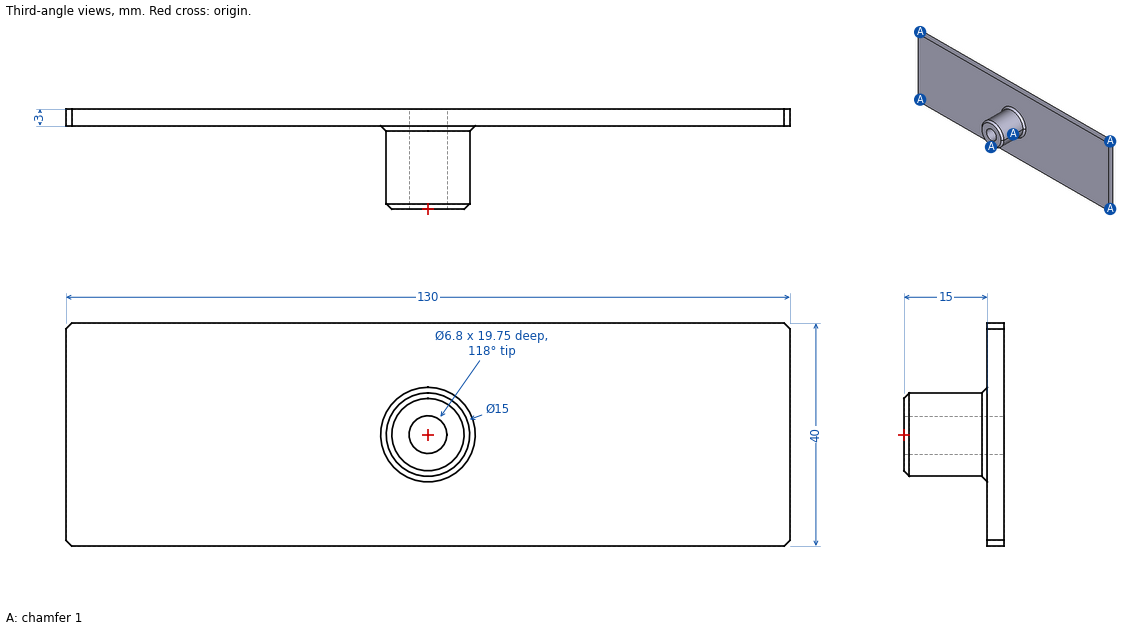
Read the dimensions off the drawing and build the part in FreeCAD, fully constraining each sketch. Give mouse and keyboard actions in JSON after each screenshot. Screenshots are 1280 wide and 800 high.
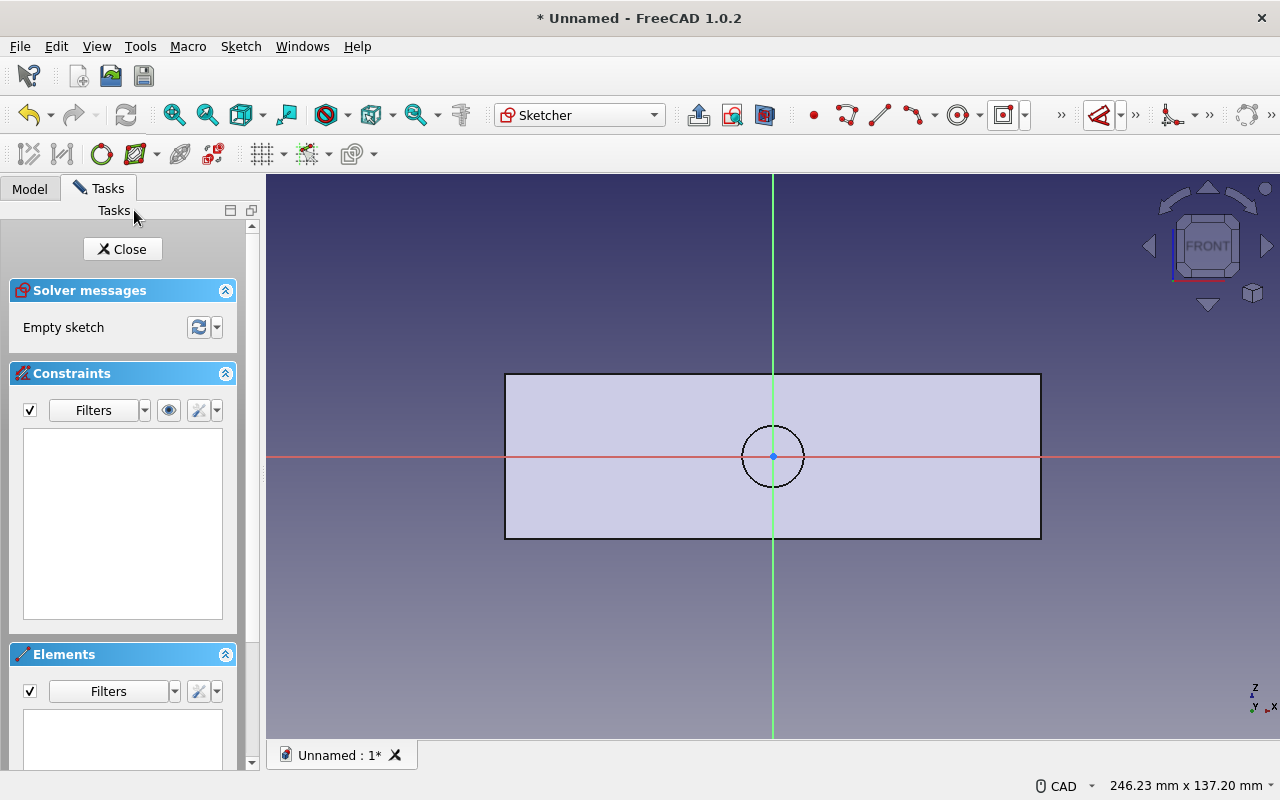
{"action": "scroll", "coordinate": [778, 457], "scroll_direction": "up", "scroll_amount": 13}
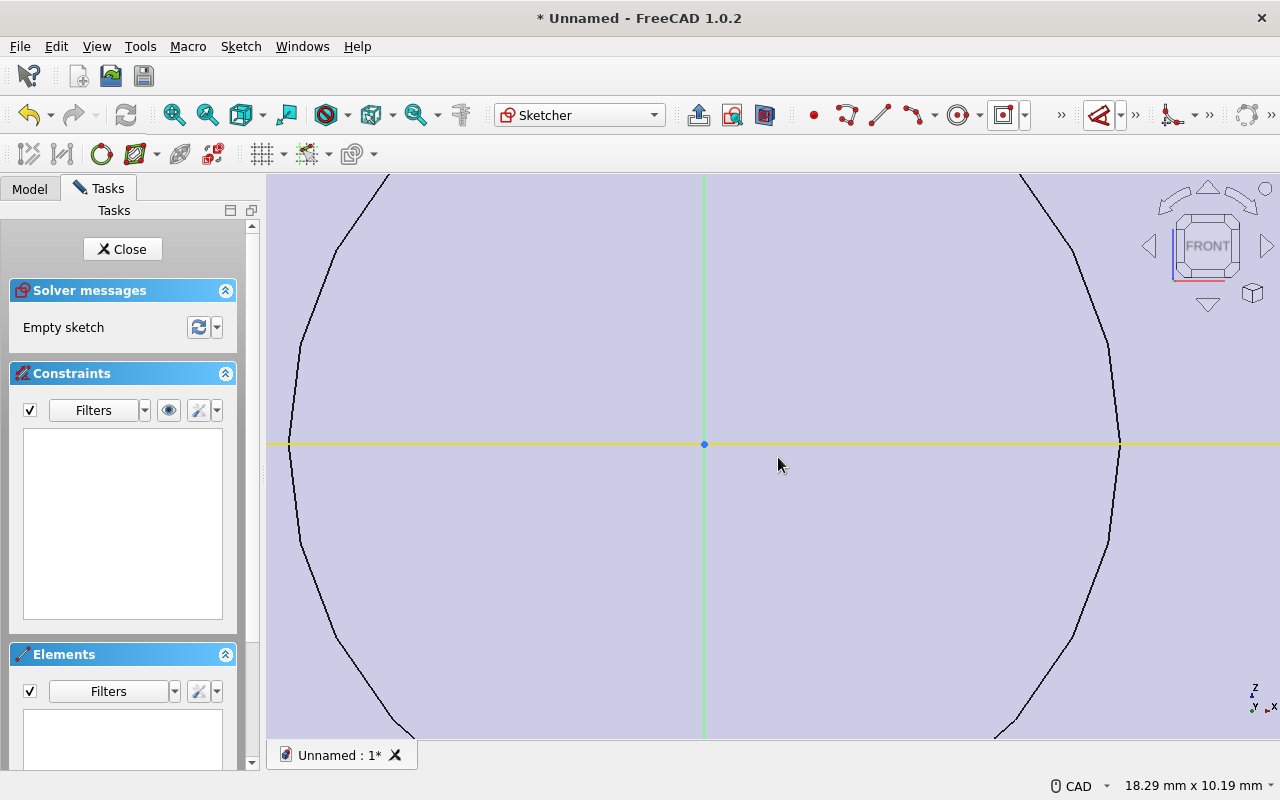
{"action": "left_click", "coordinate": [958, 116]}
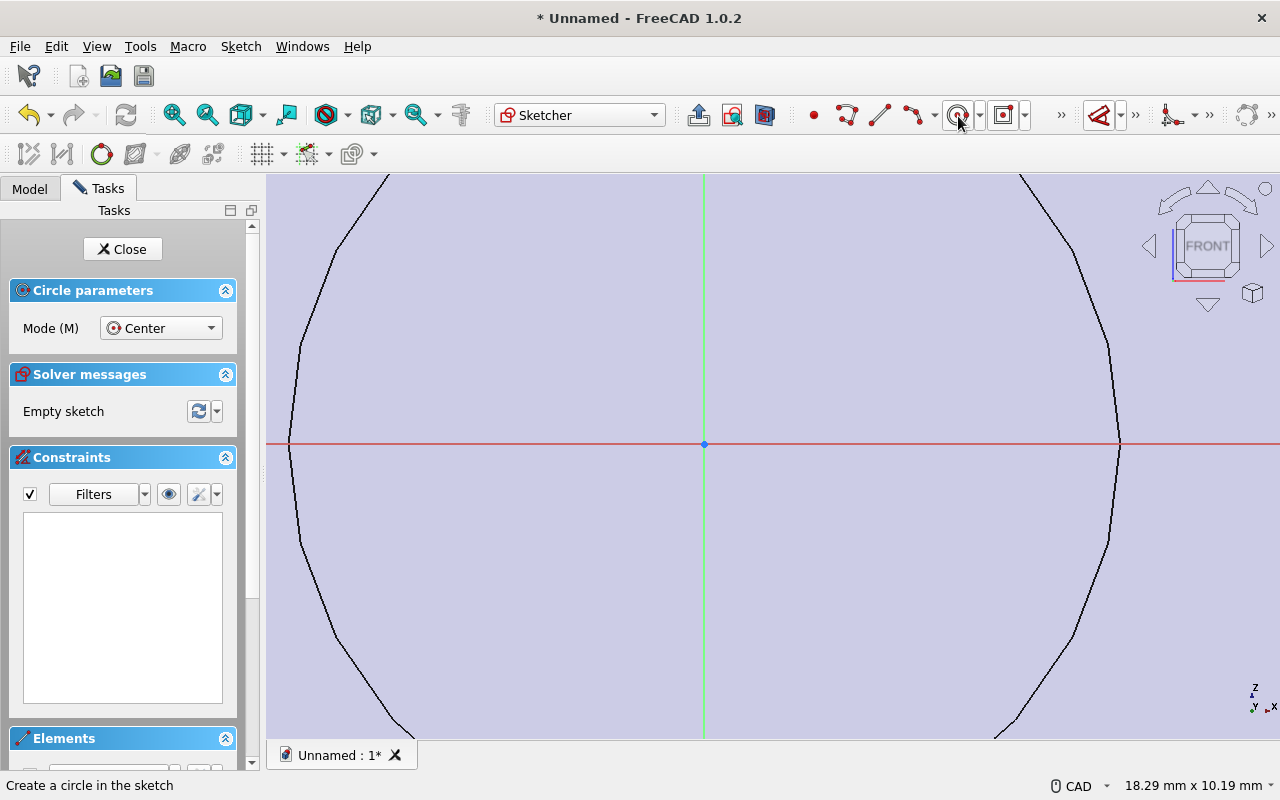
{"action": "left_click", "coordinate": [704, 444]}
{"action": "mouse_move", "coordinate": [838, 311]}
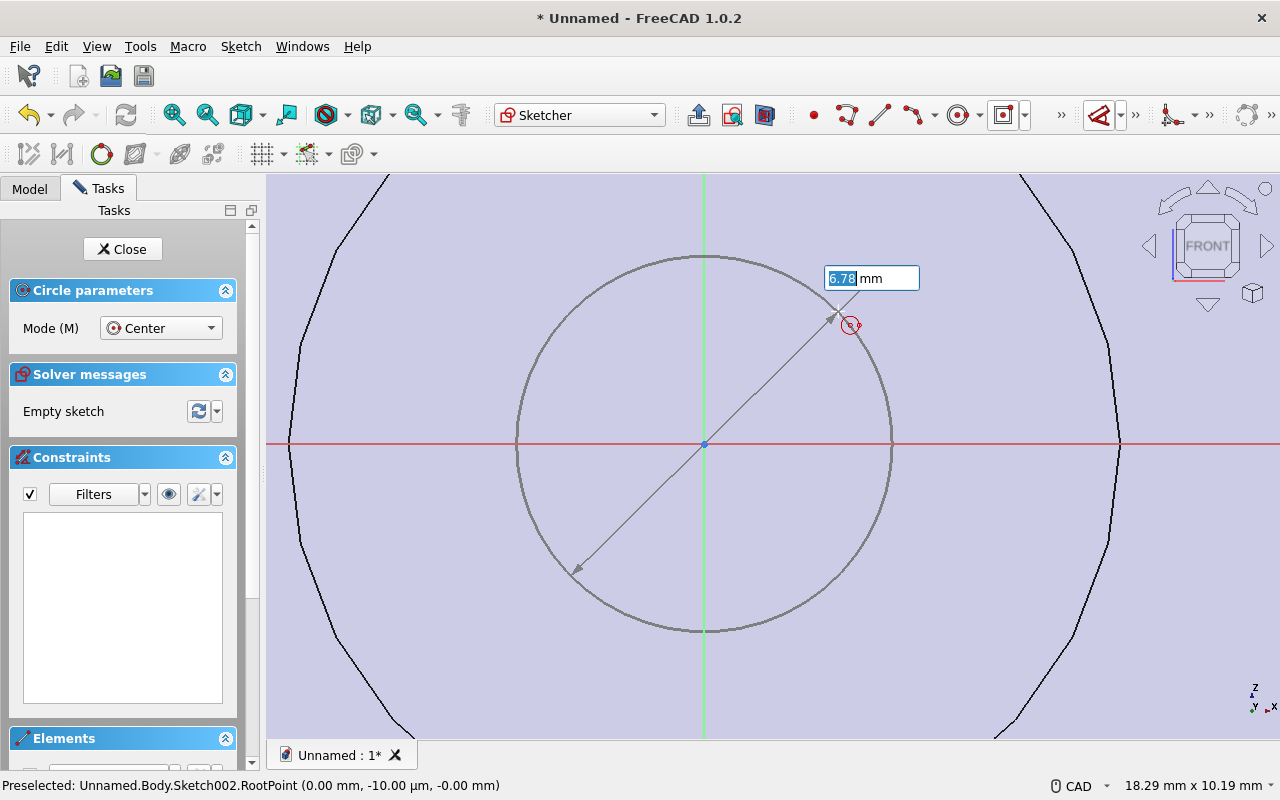
{"action": "type", "text": "6.8"}
{"action": "key", "text": "Return"}
{"action": "key", "text": "Escape"}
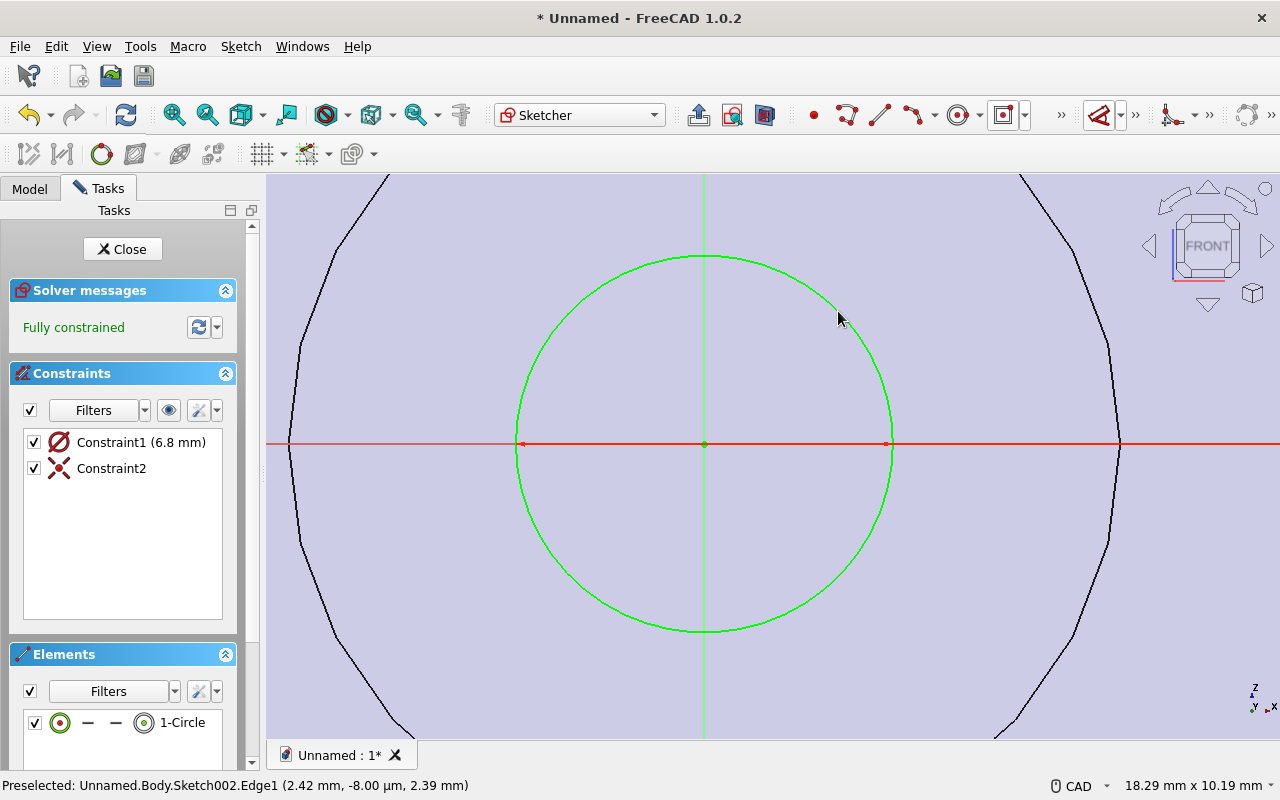
{"action": "left_click", "coordinate": [123, 249]}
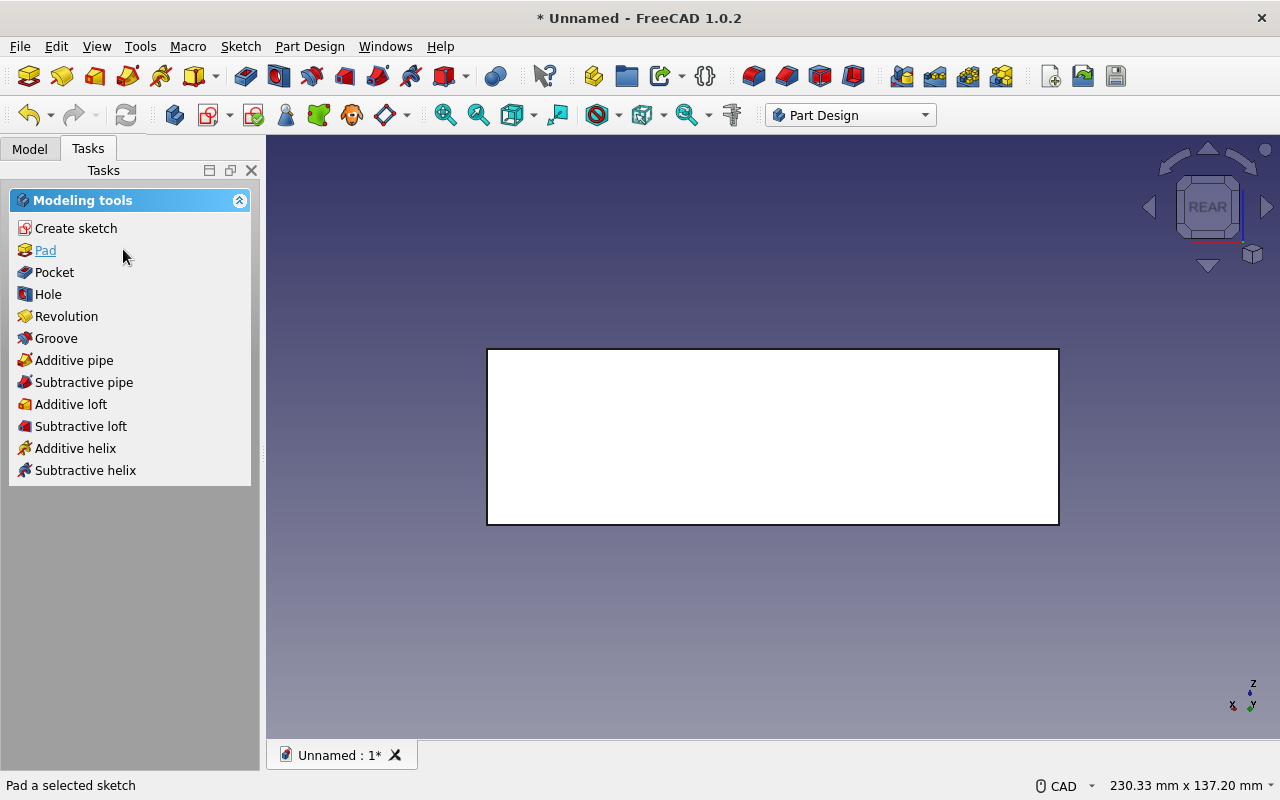
{"action": "left_click", "coordinate": [279, 76]}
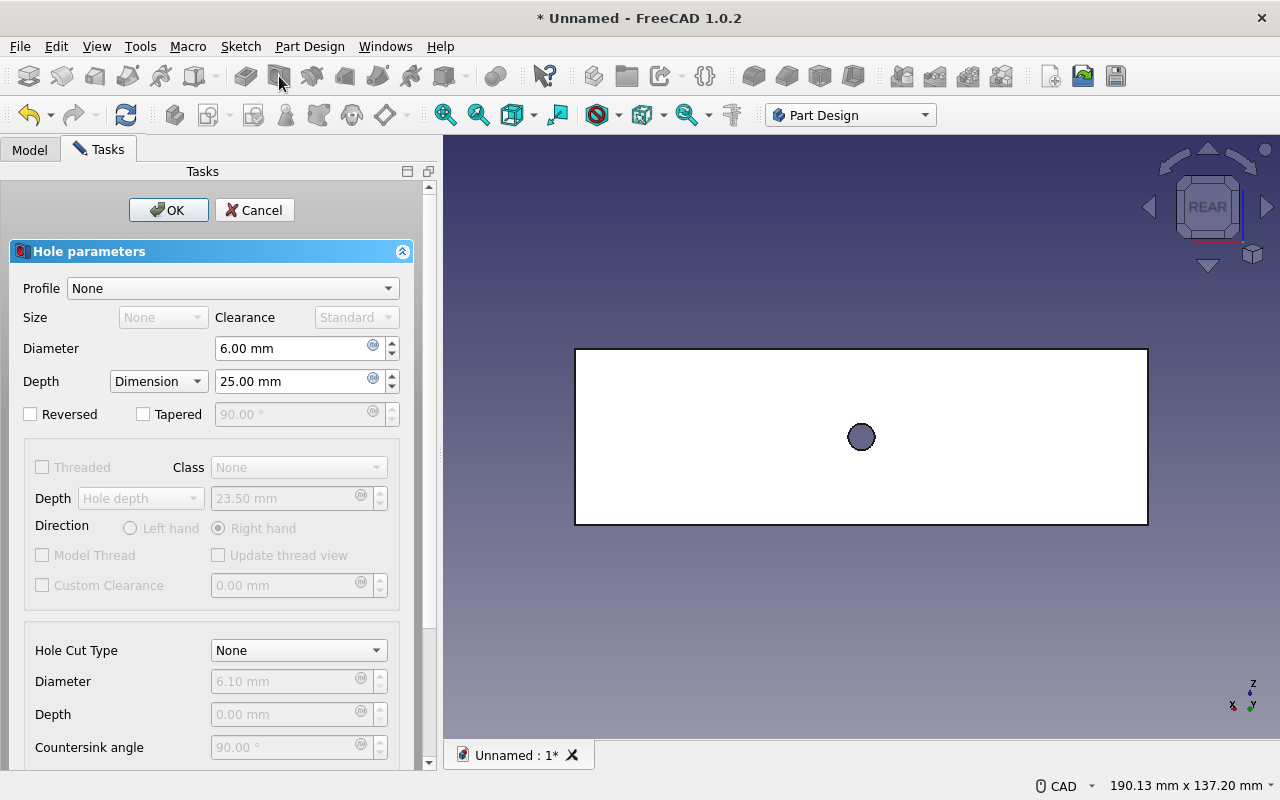
{"action": "triple_click", "coordinate": [300, 348]}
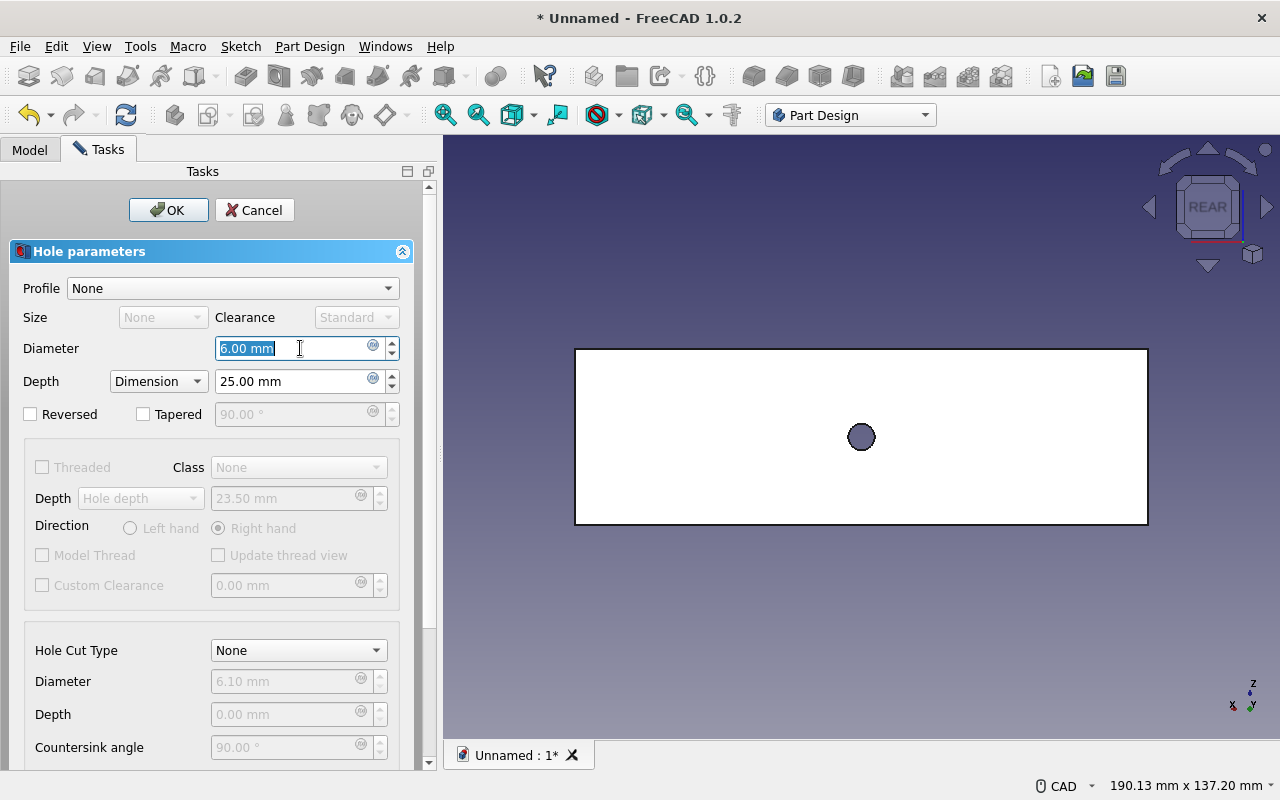
{"action": "type", "text": "6.8"}
{"action": "key", "text": "Tab"}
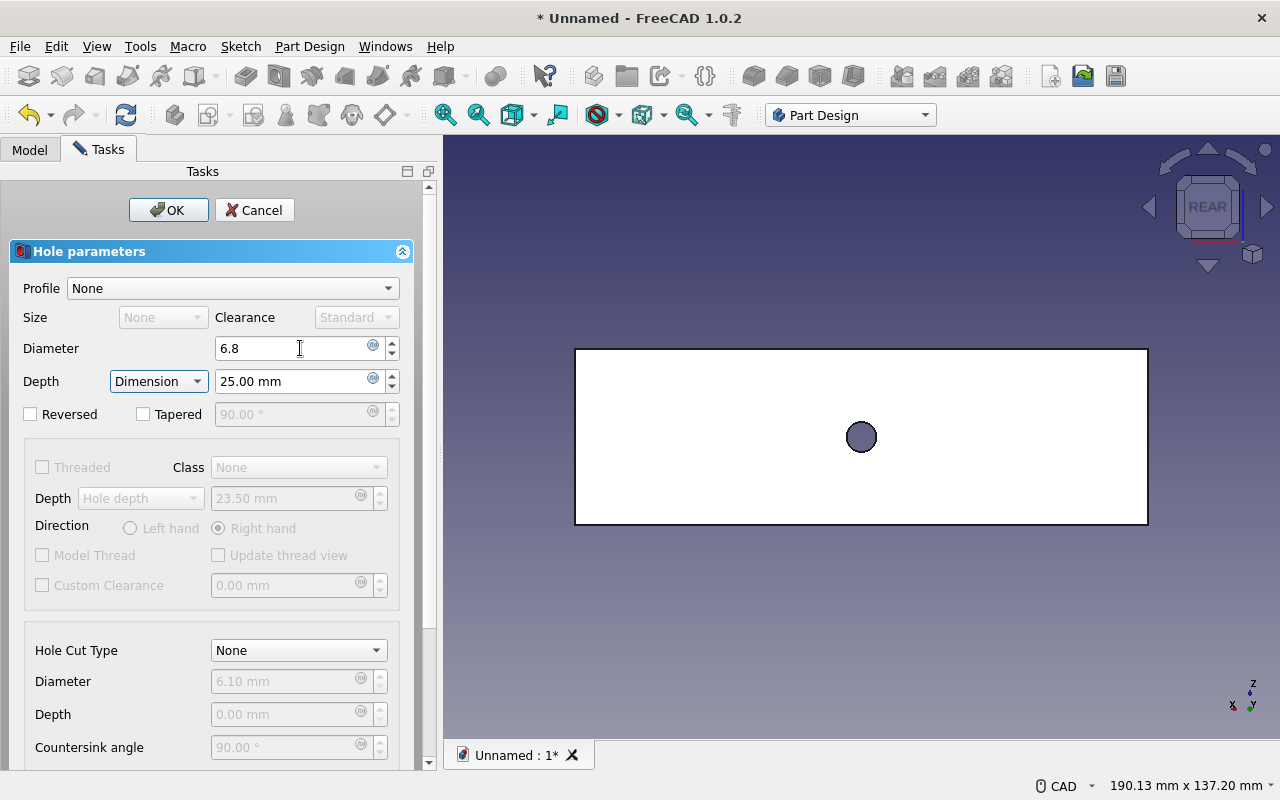
{"action": "triple_click", "coordinate": [300, 382]}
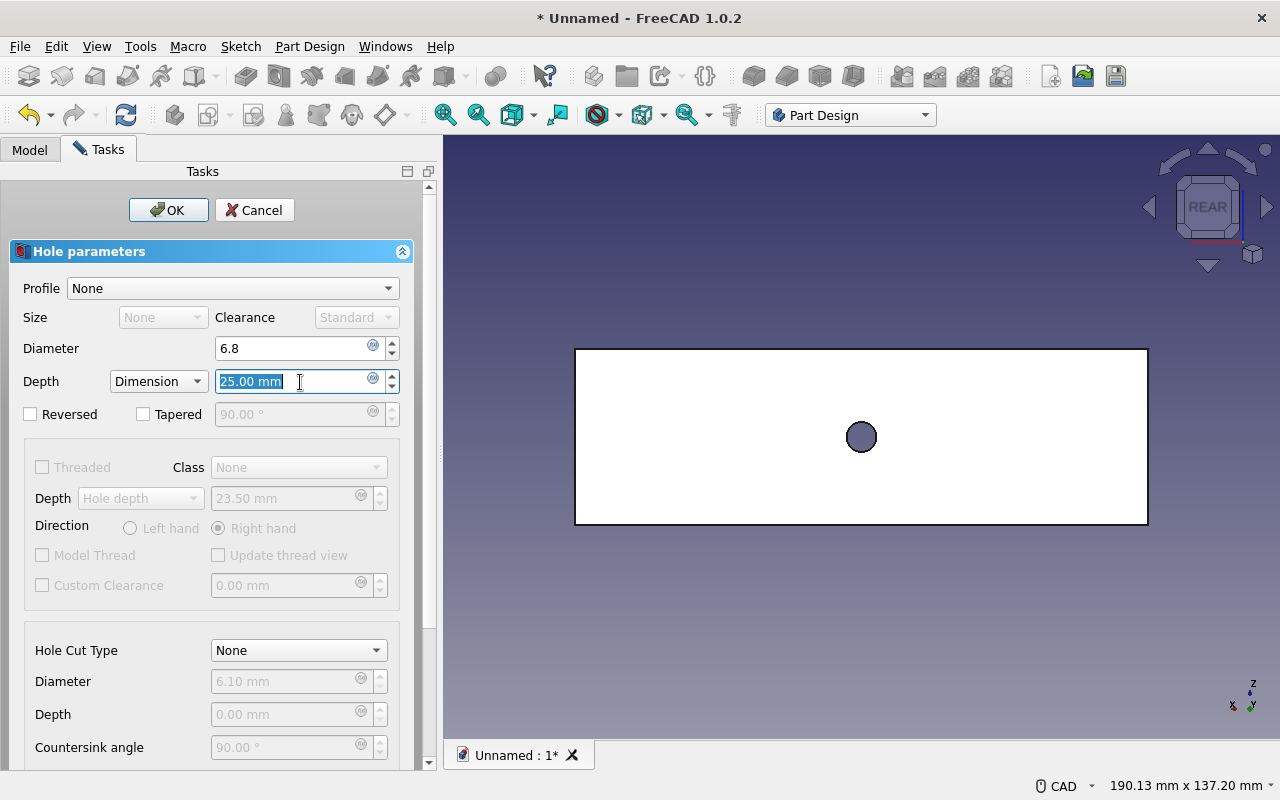
{"action": "type", "text": "19.75"}
{"action": "key", "text": "Tab"}